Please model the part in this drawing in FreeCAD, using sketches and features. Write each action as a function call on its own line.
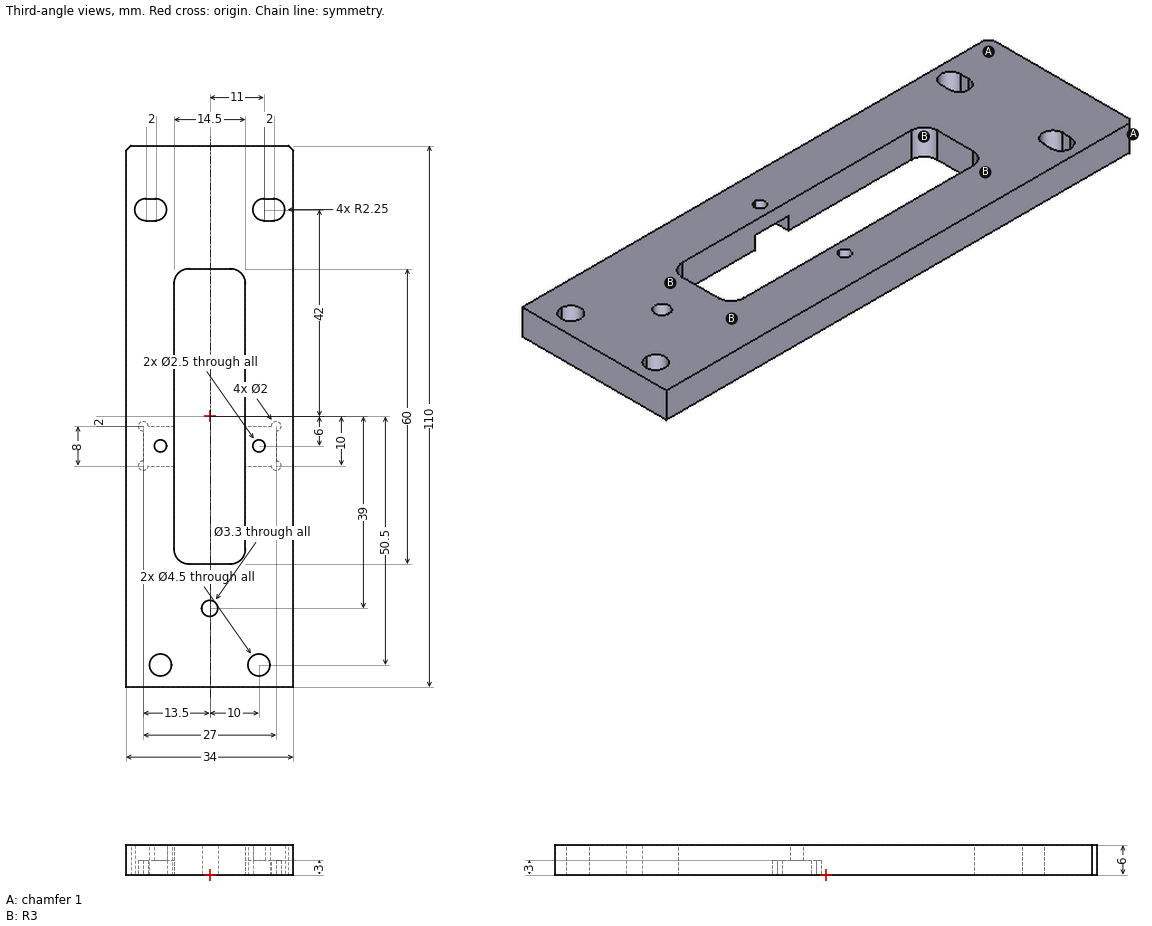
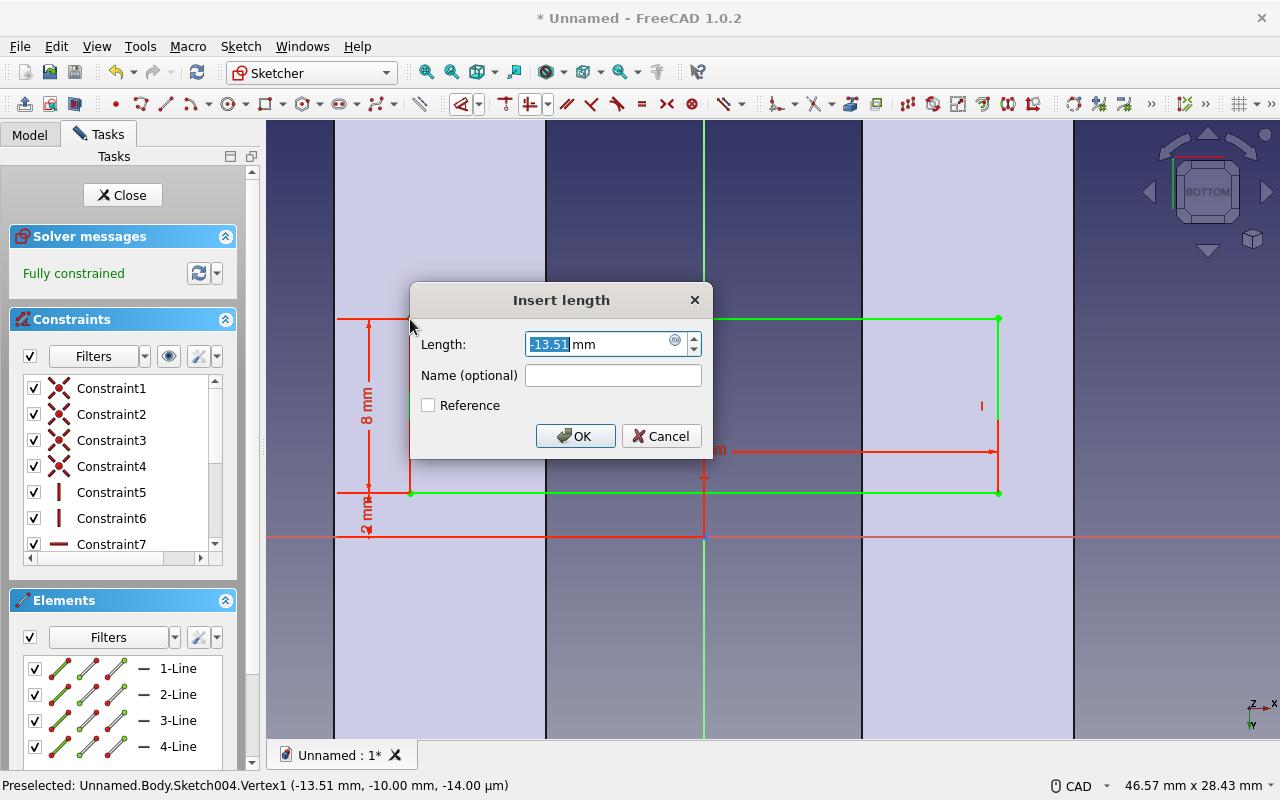
text(-13.5)
key(Return)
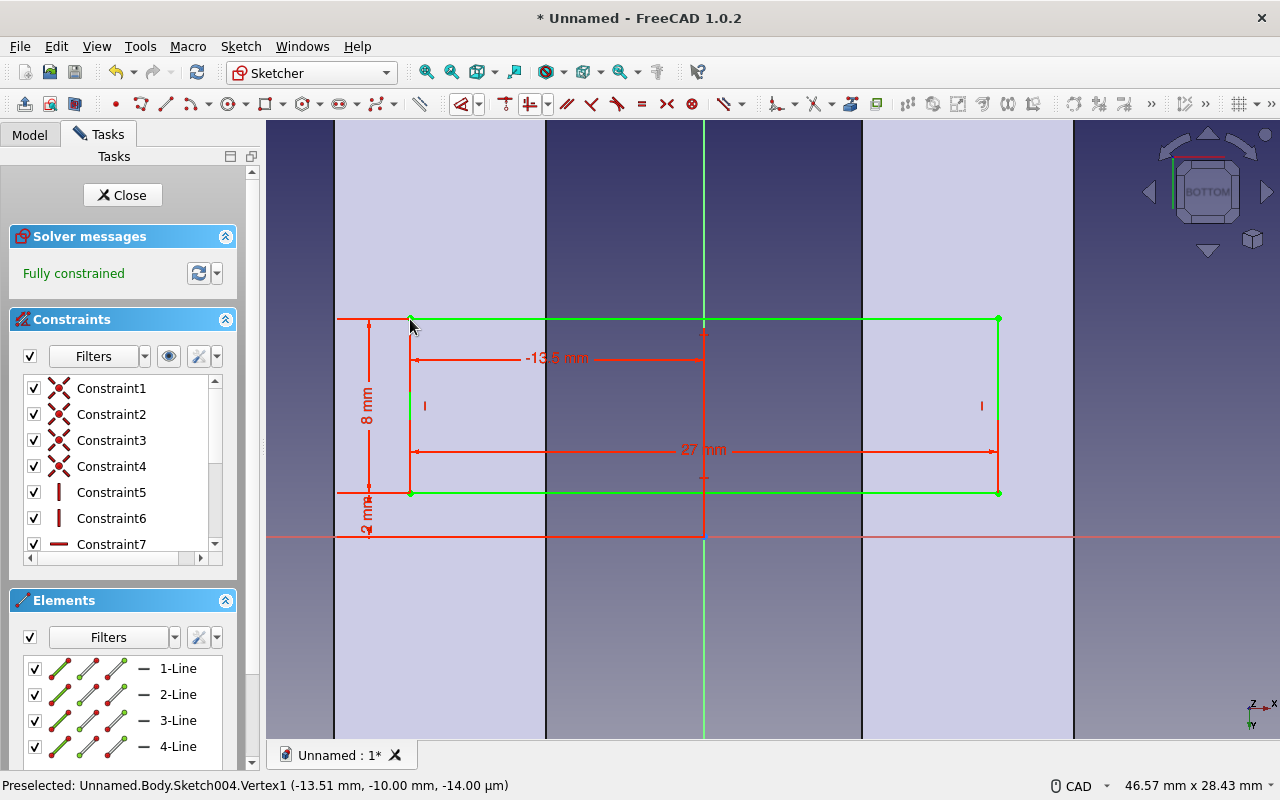
click(123, 195)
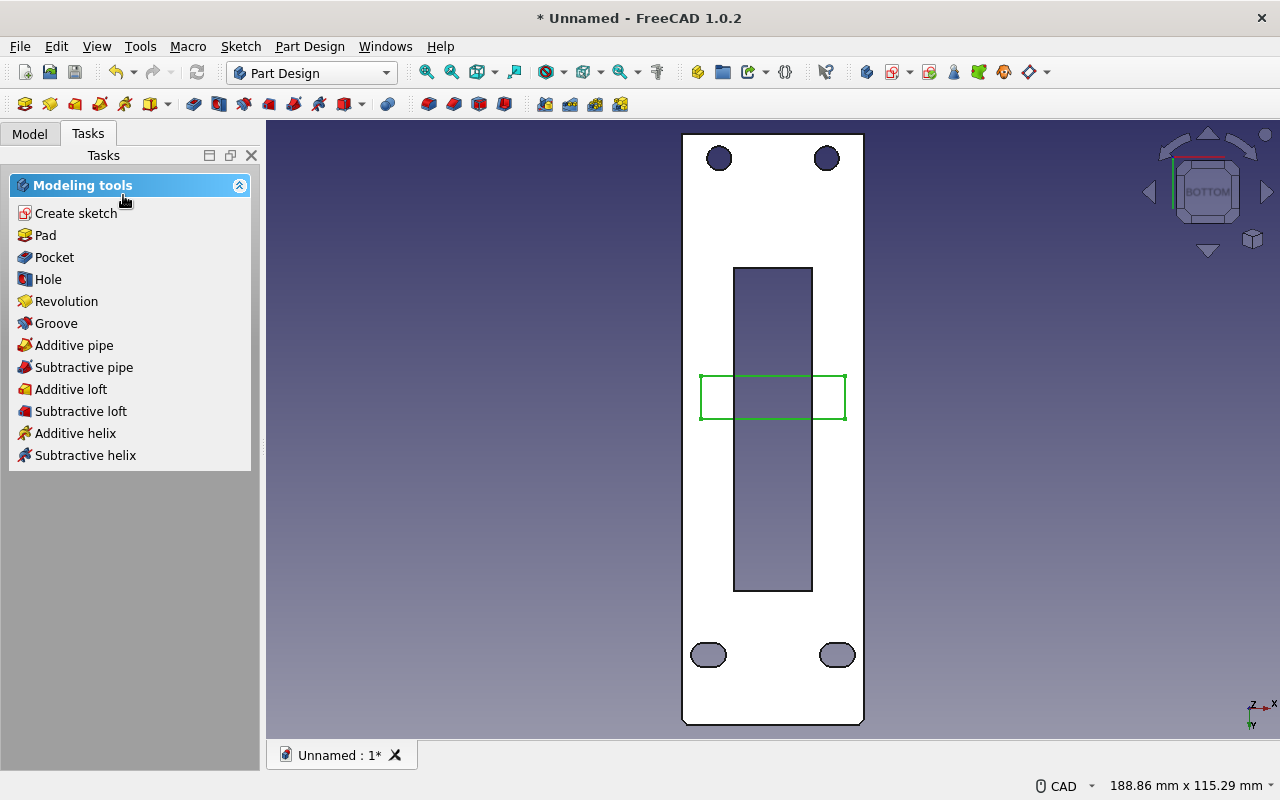
click(194, 104)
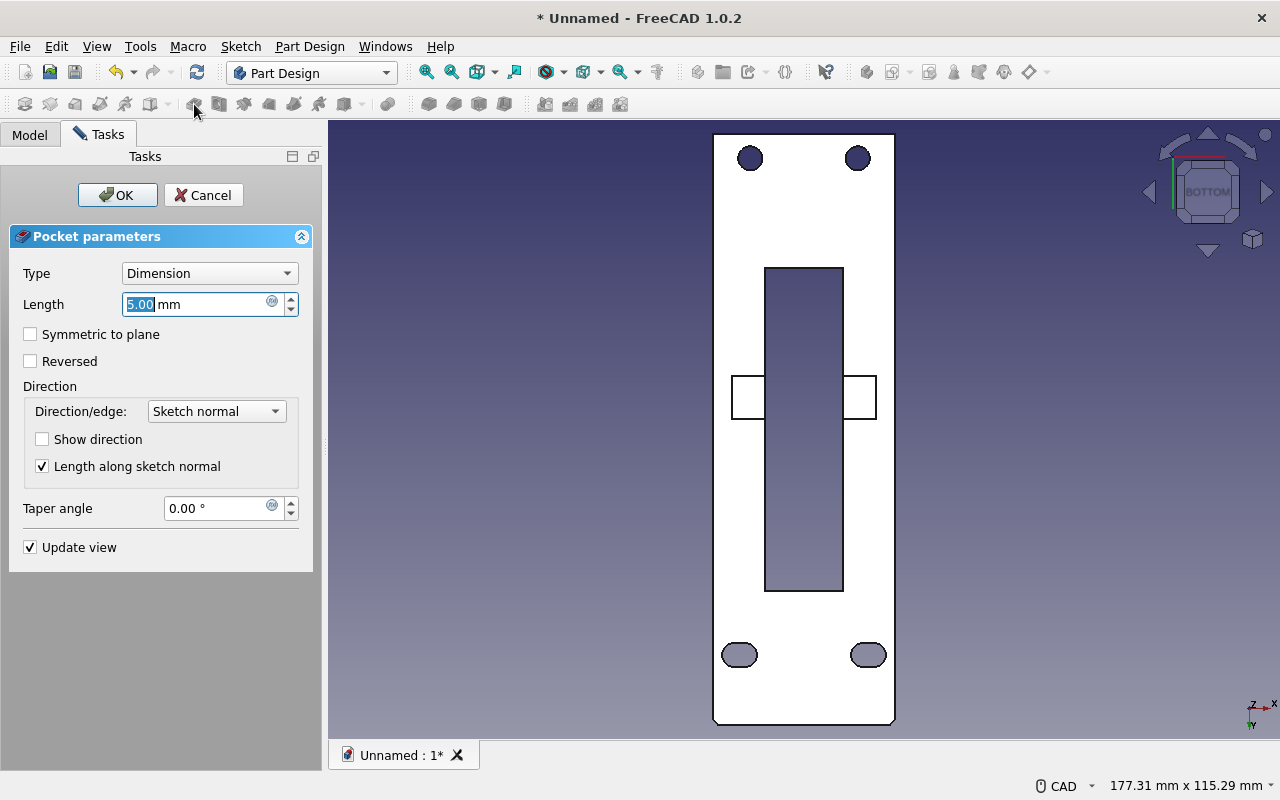
text(3)
key(Tab)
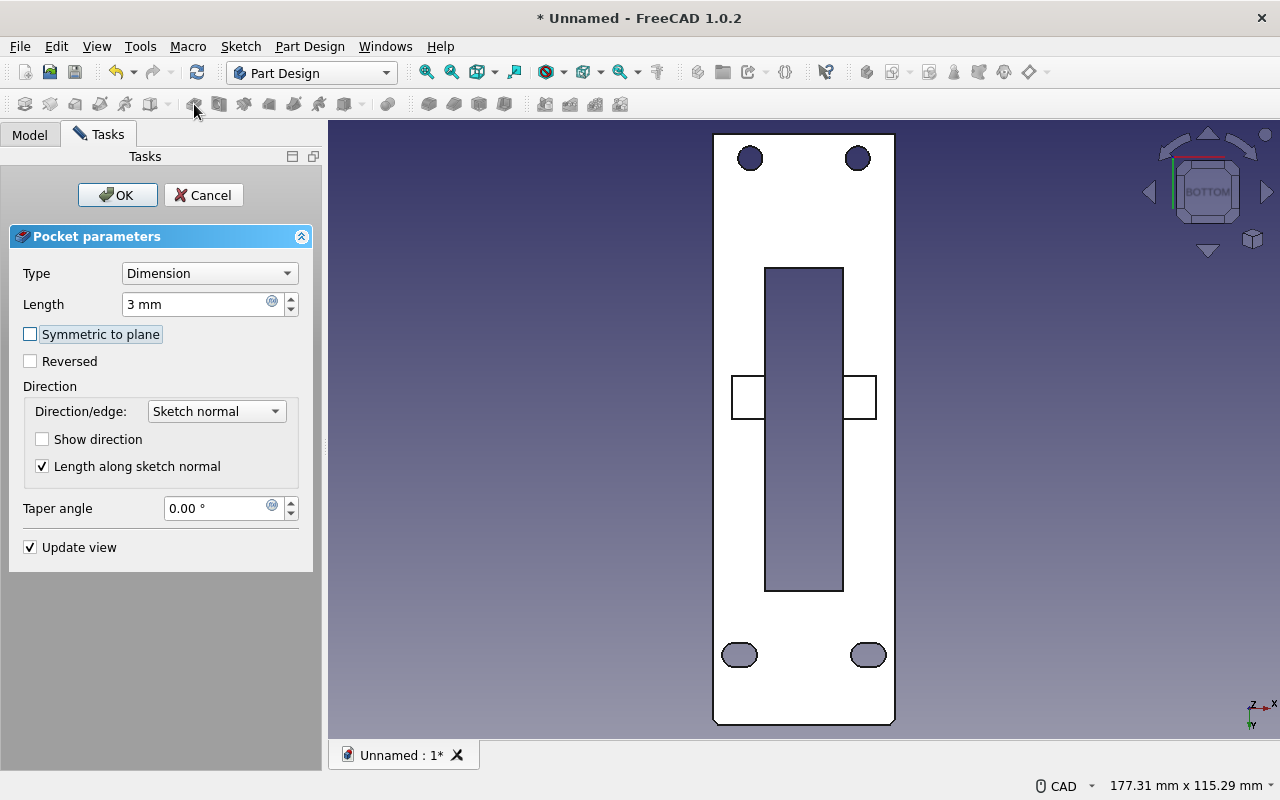
click(118, 195)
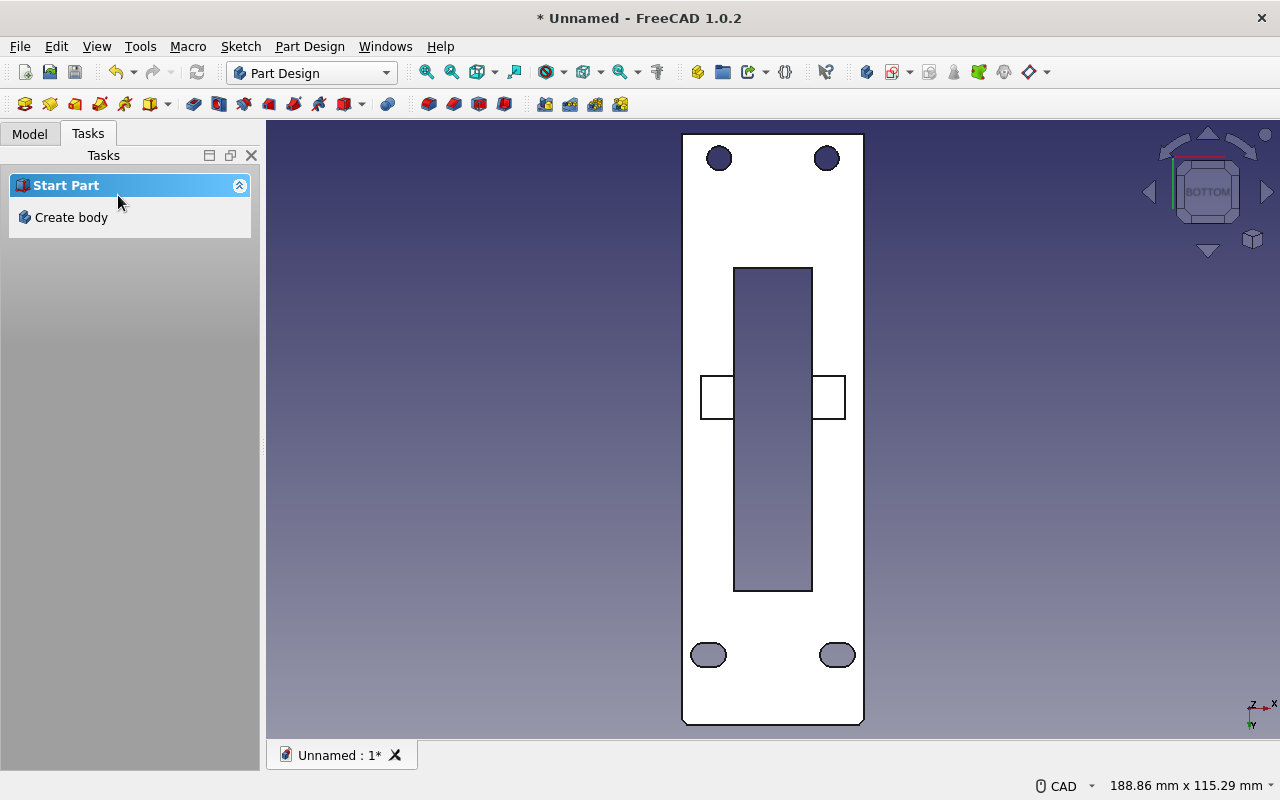
key(0)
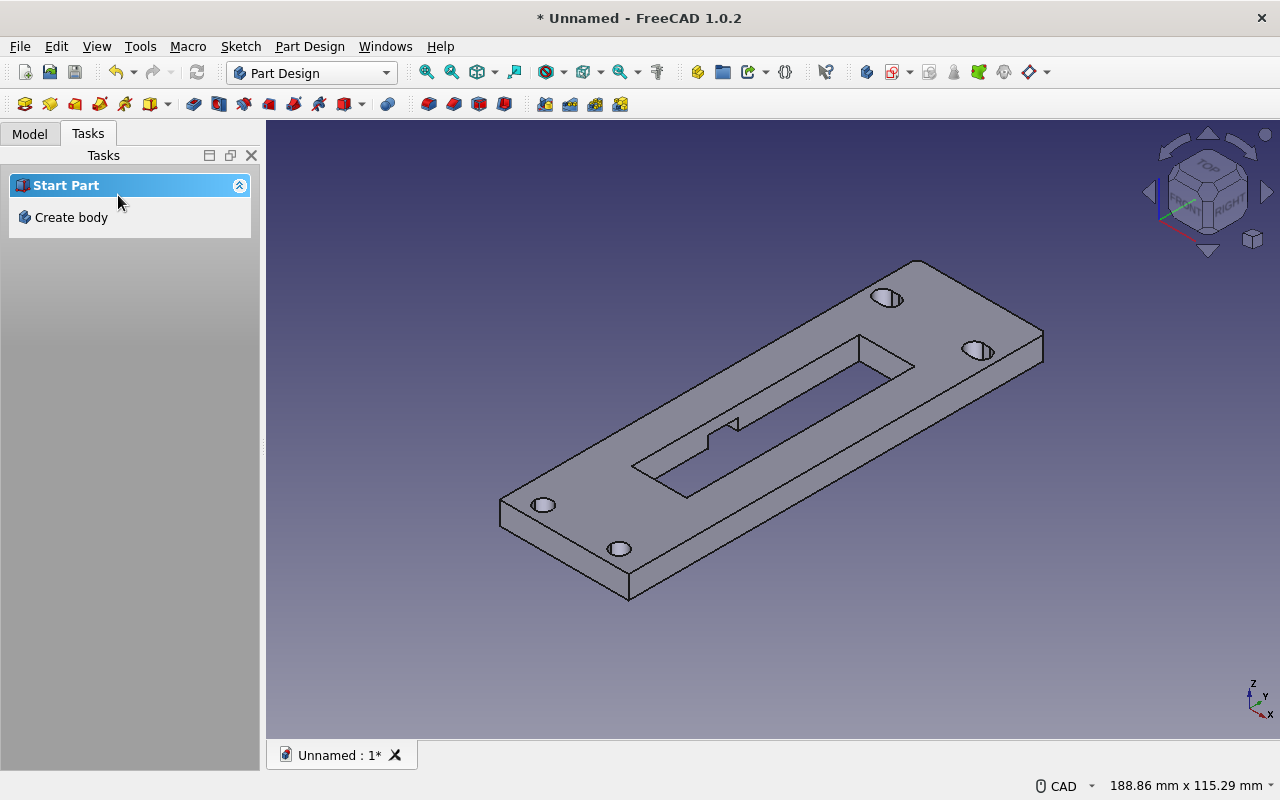
key(2)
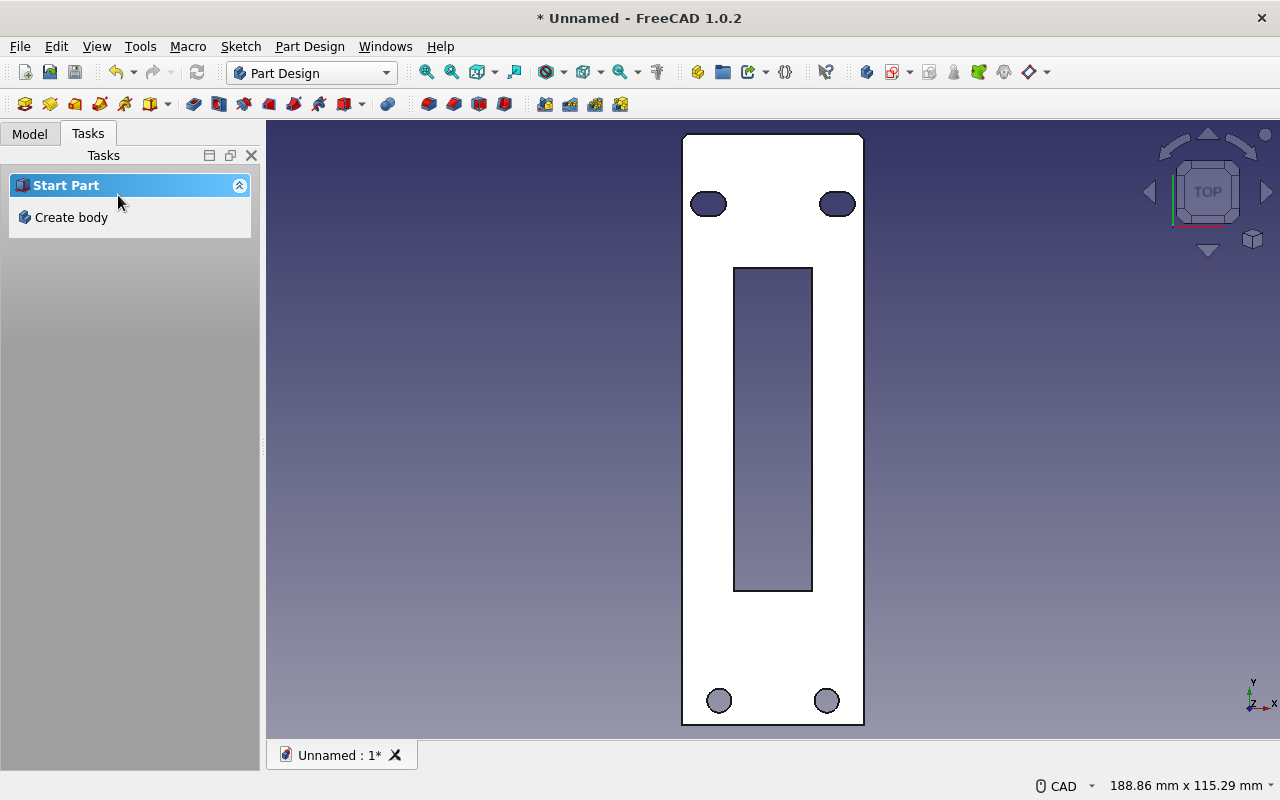
key(1)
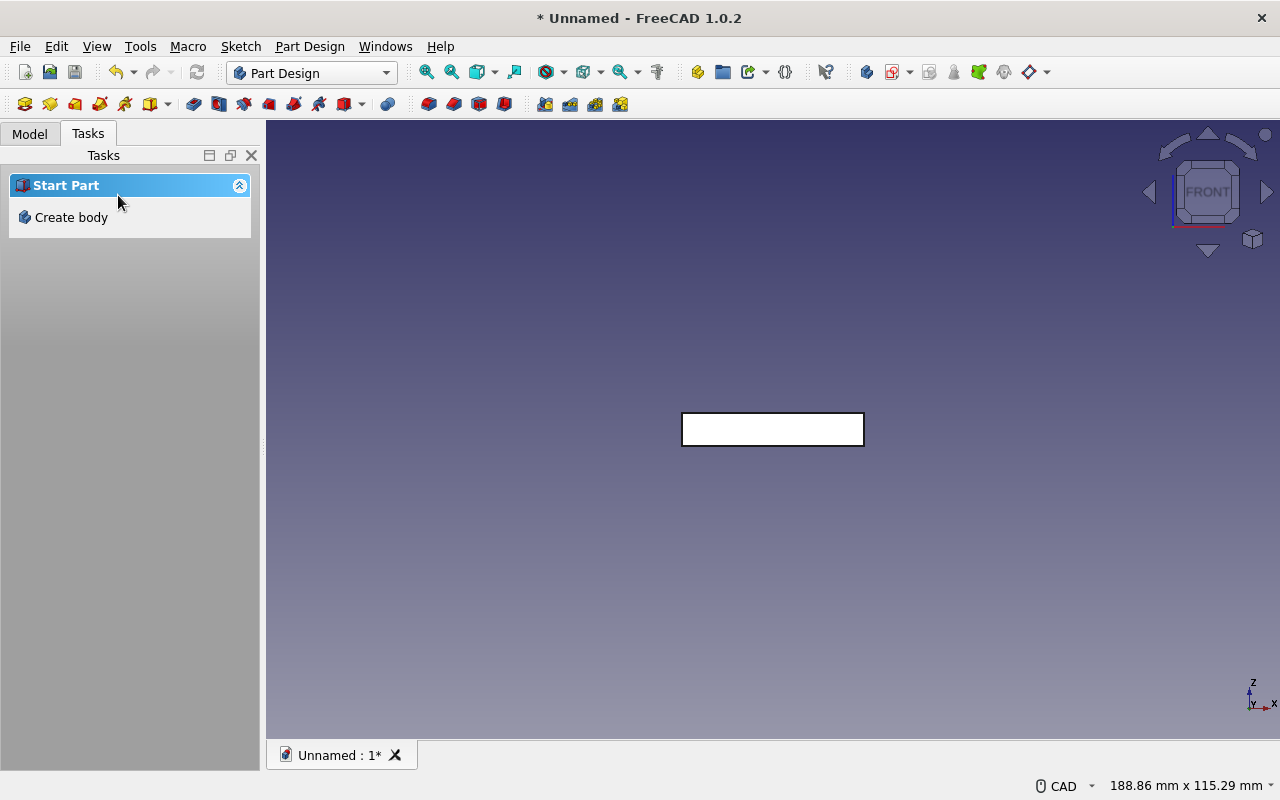
key(v)
key(f)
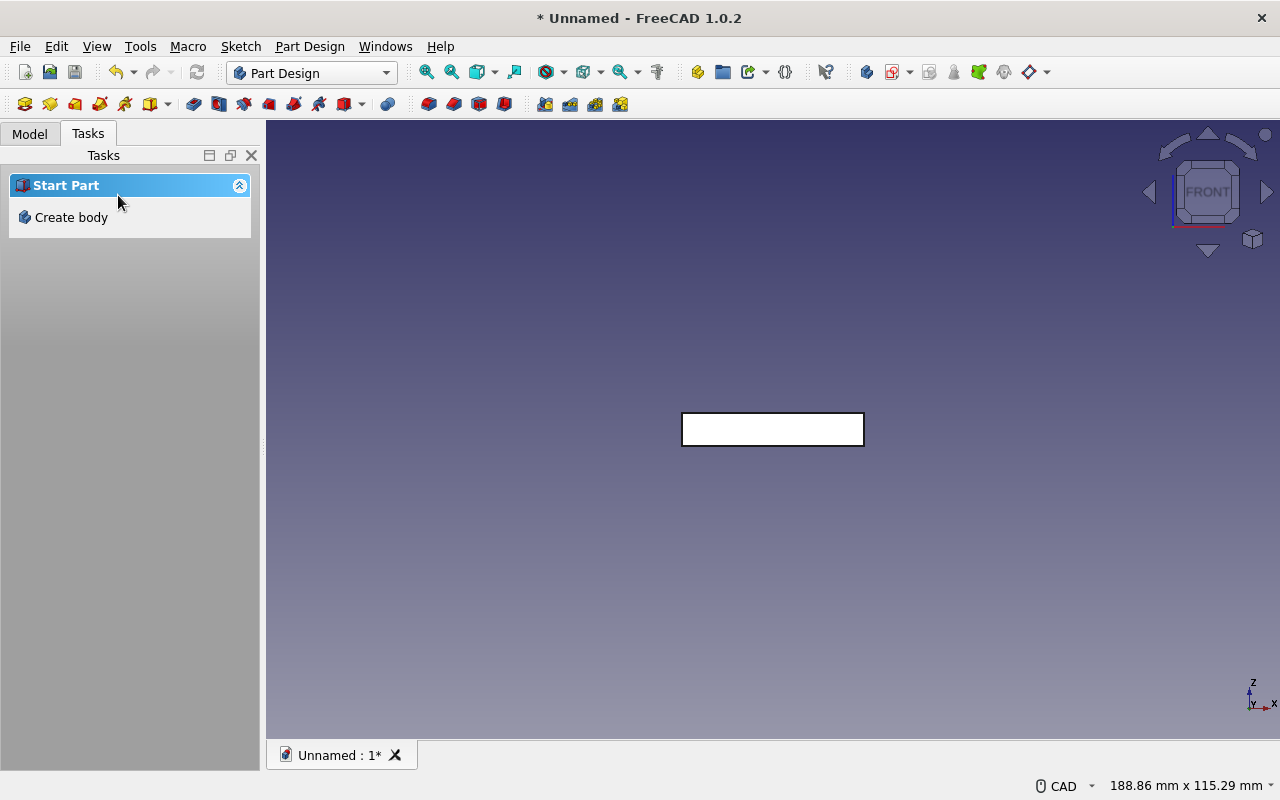
key(3)